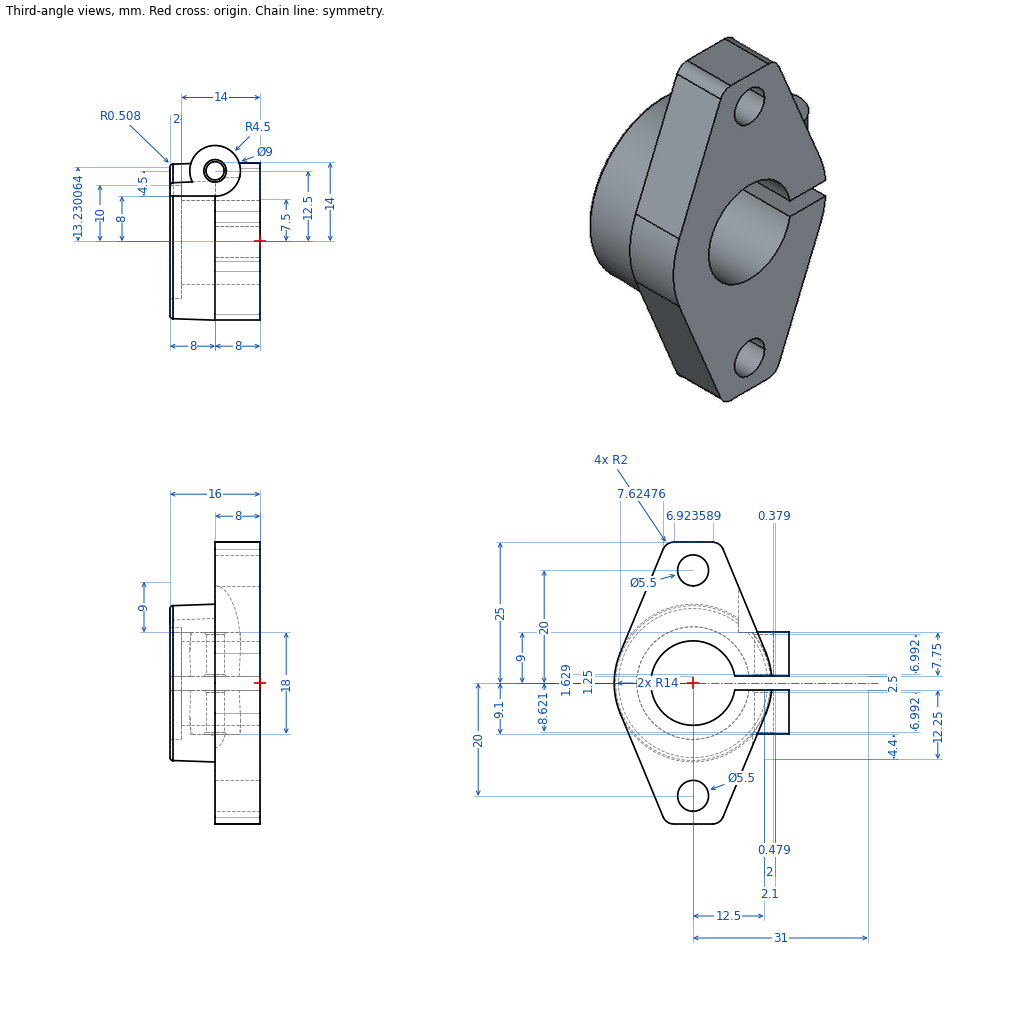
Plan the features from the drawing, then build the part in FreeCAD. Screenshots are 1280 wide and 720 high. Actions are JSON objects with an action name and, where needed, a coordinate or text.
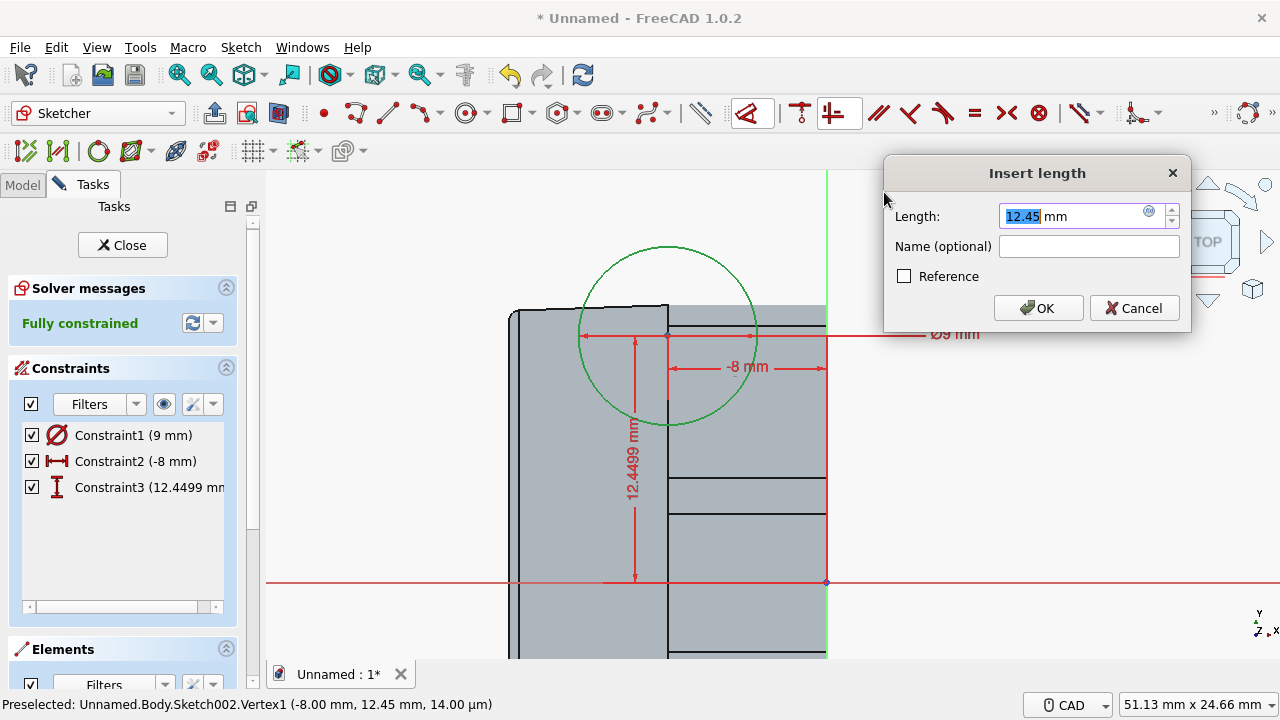
{"action": "type", "text": "12.5"}
{"action": "key", "text": "Return"}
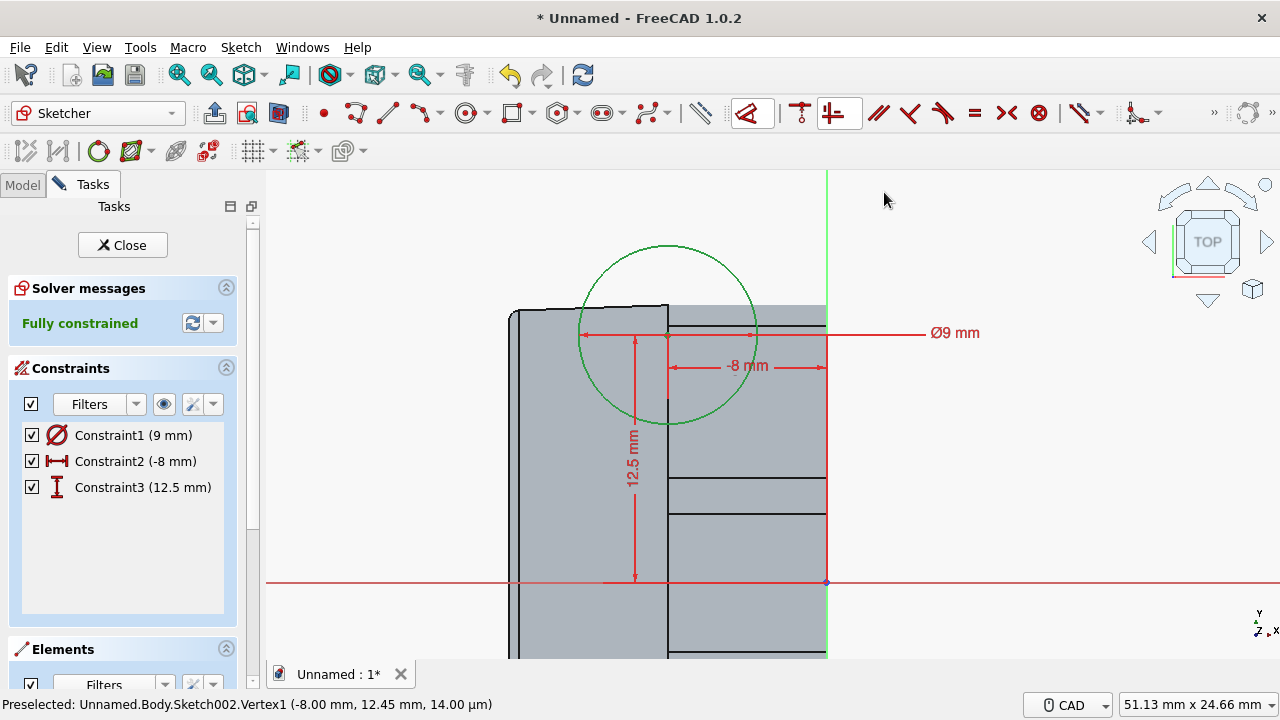
{"action": "left_click", "coordinate": [123, 245]}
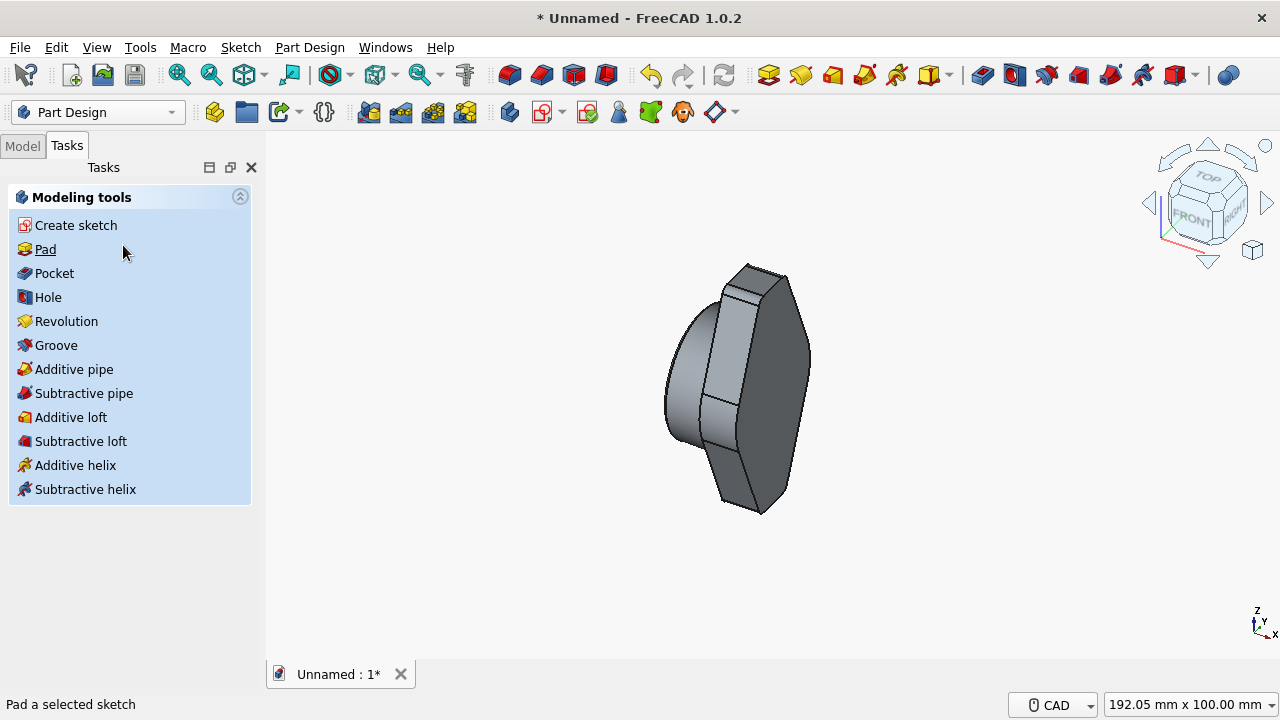
{"action": "left_click", "coordinate": [770, 76]}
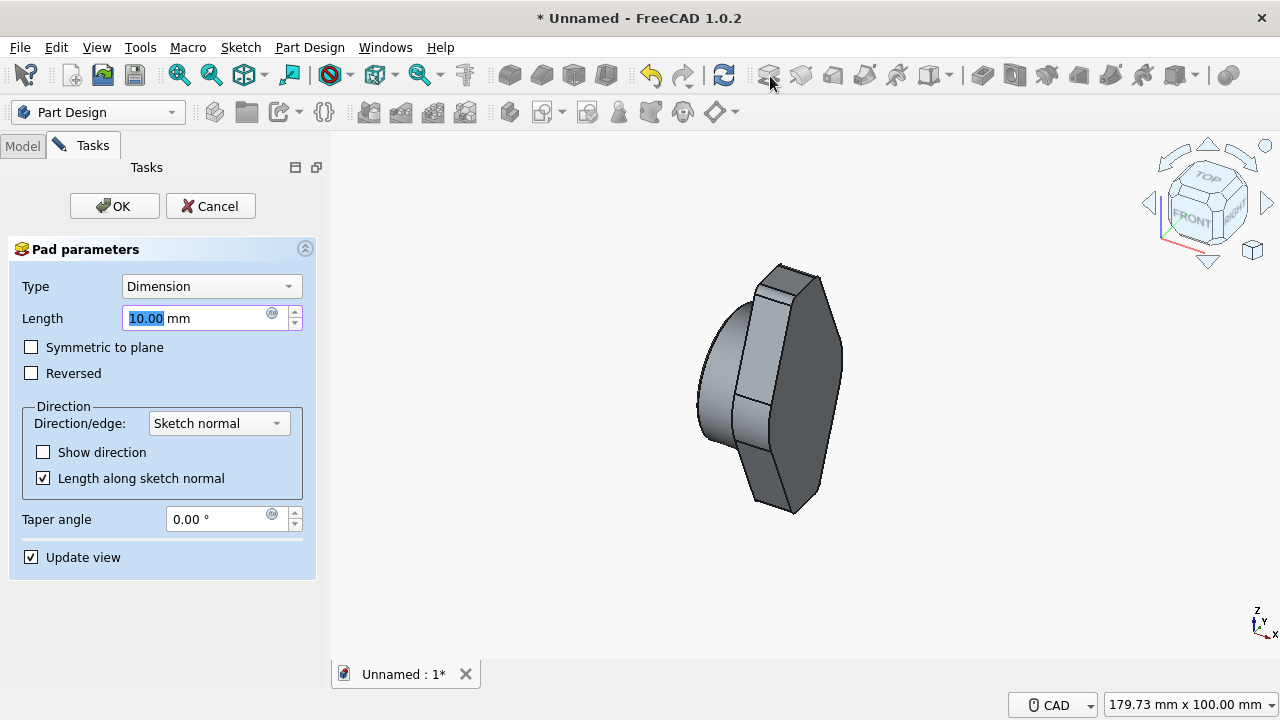
{"action": "type", "text": "18"}
{"action": "key", "text": "Tab"}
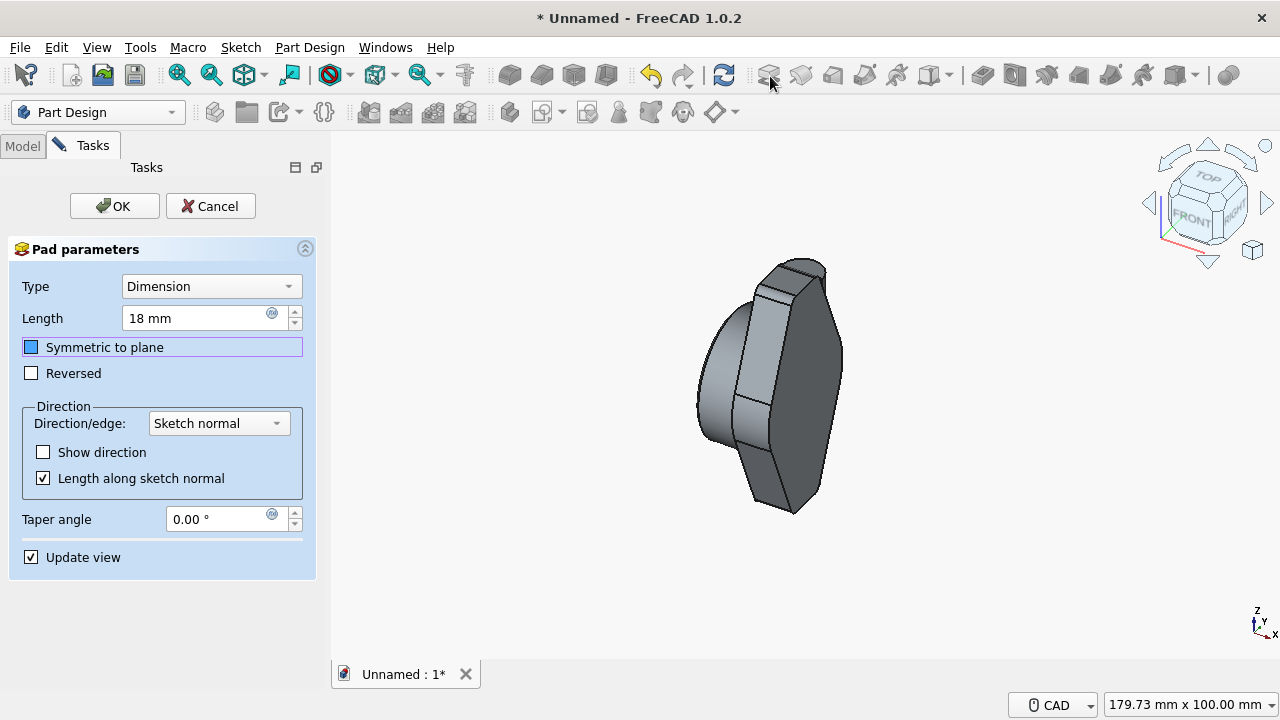
{"action": "left_click", "coordinate": [30, 347]}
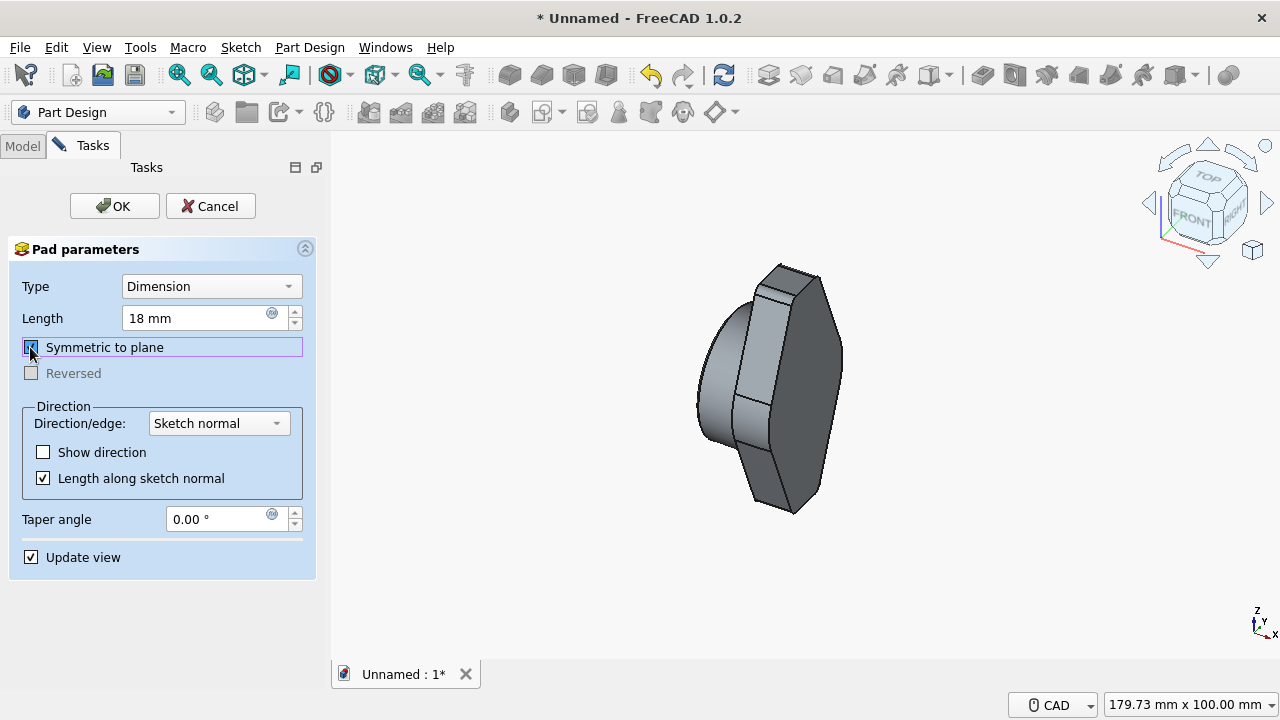
{"action": "left_click", "coordinate": [115, 206]}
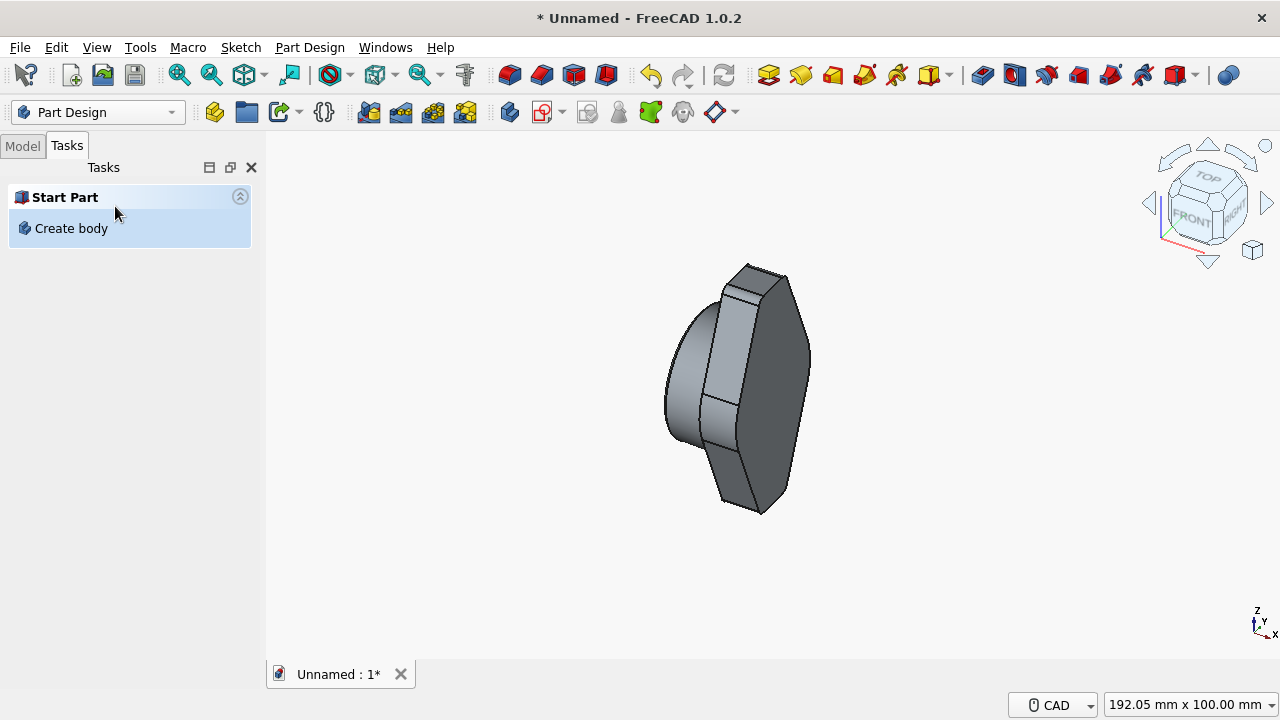
{"action": "key", "text": "0"}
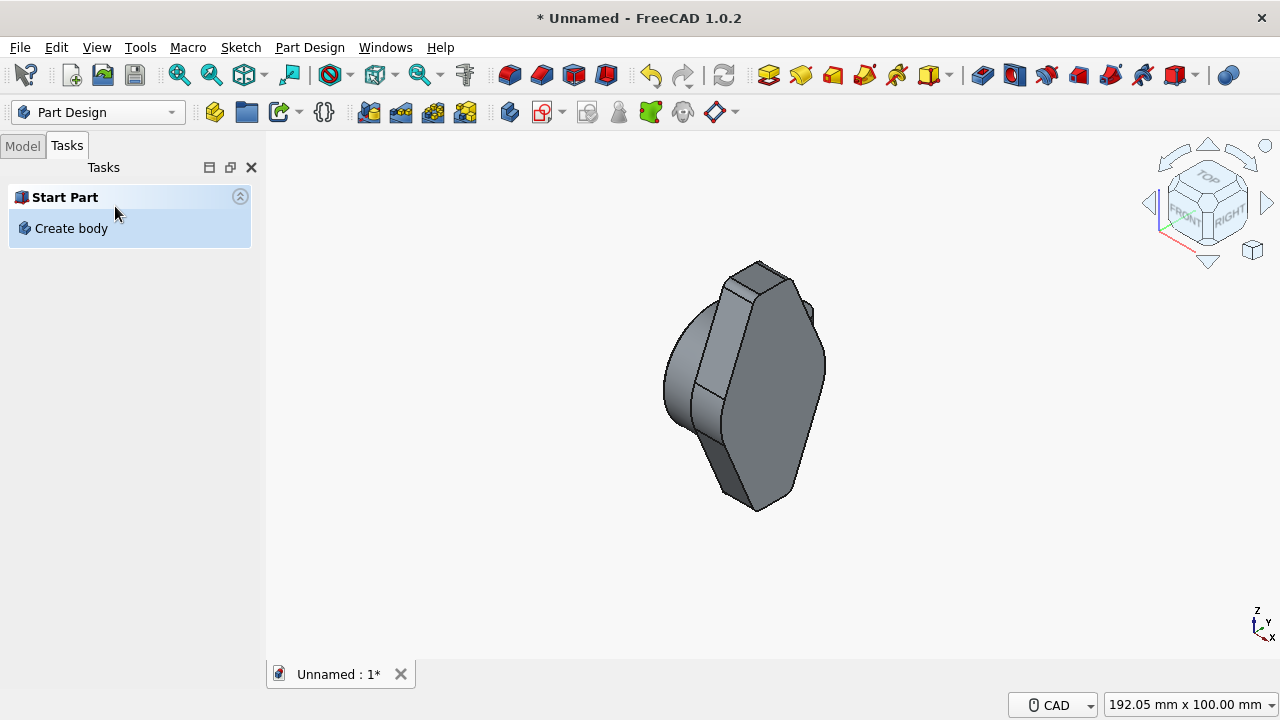
{"action": "key", "text": "2"}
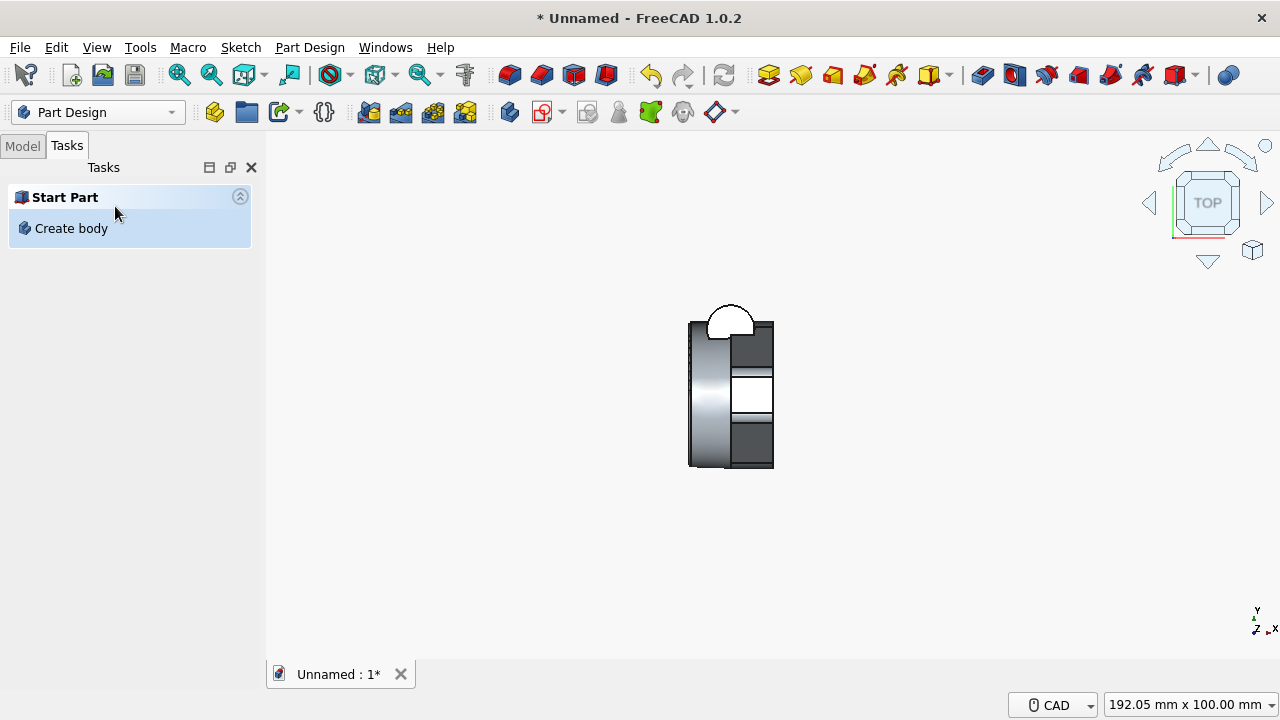
{"action": "left_click", "coordinate": [180, 76]}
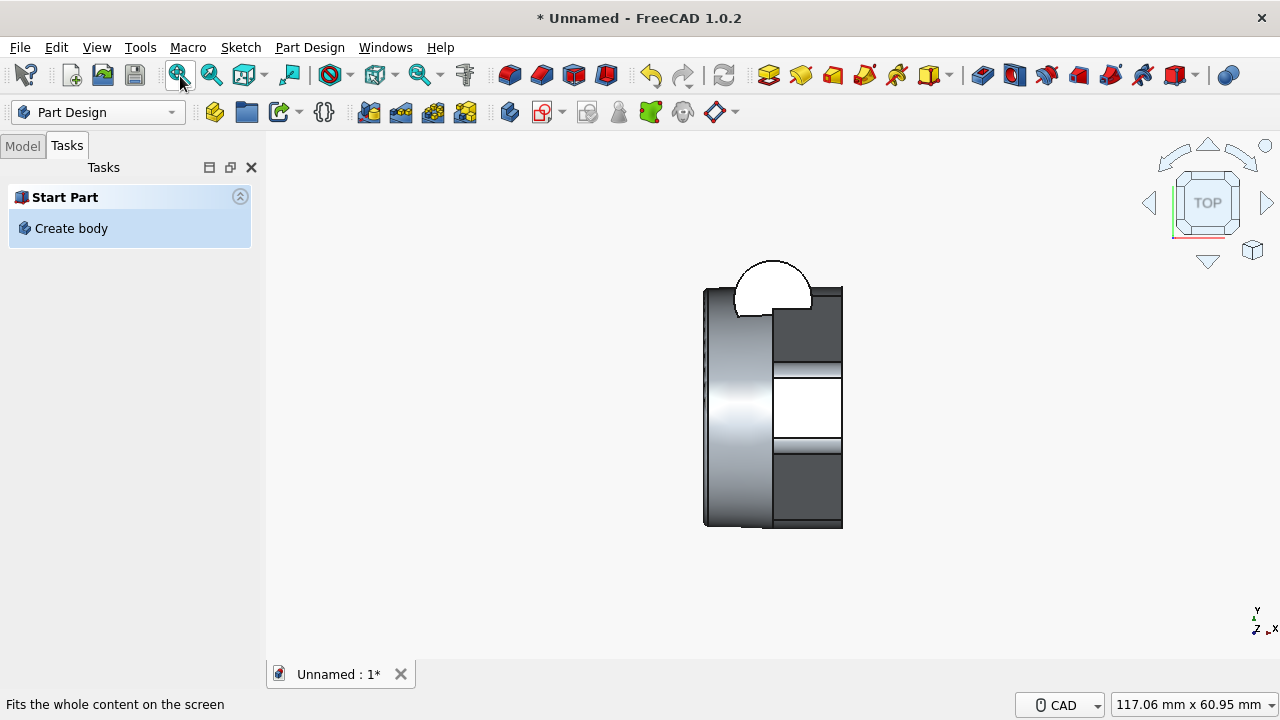
{"action": "left_click", "coordinate": [762, 288]}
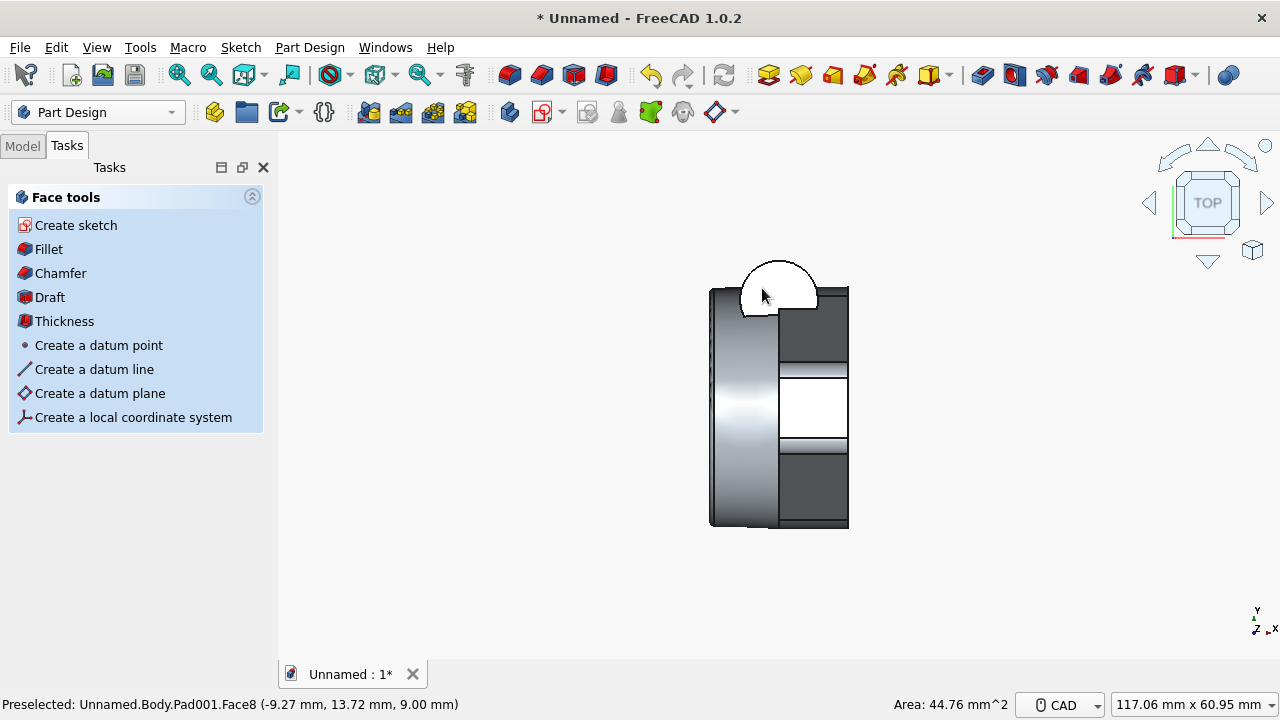
{"action": "left_click", "coordinate": [542, 112]}